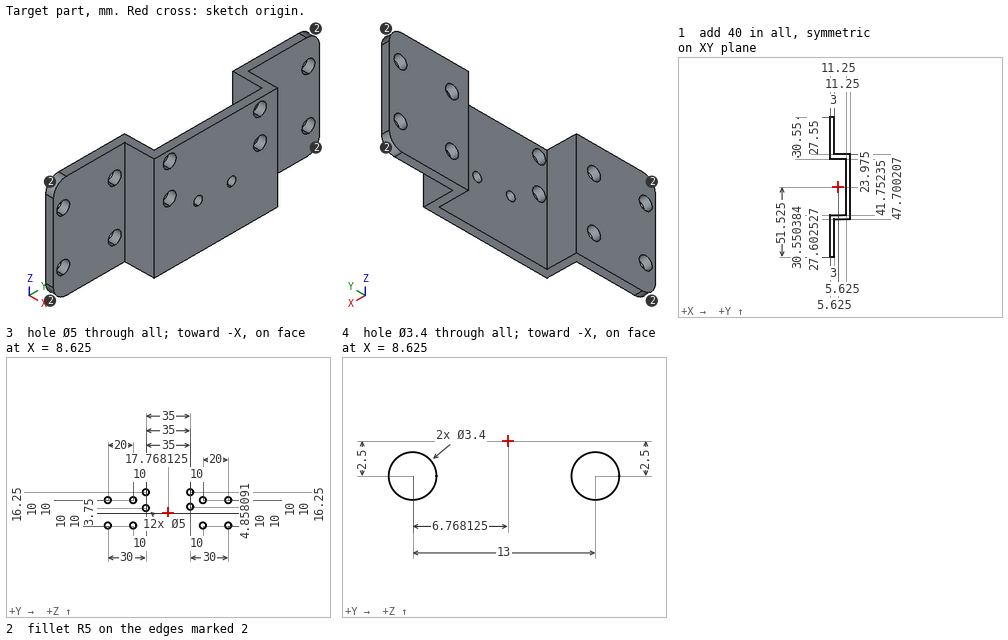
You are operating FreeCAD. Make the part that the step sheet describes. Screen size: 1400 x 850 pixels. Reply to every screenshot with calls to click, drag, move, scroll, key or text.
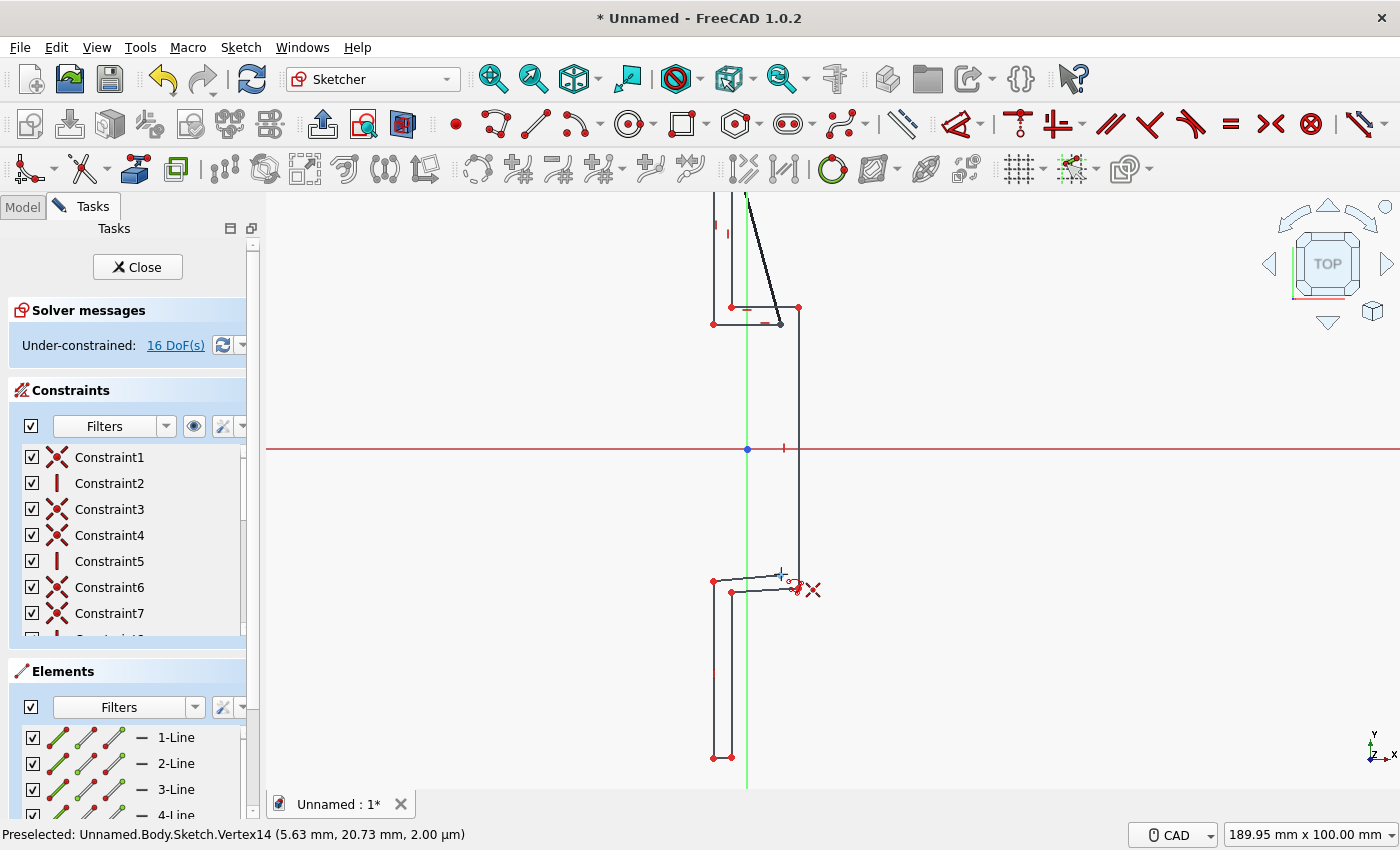
click(781, 575)
key(Escape)
key(Escape)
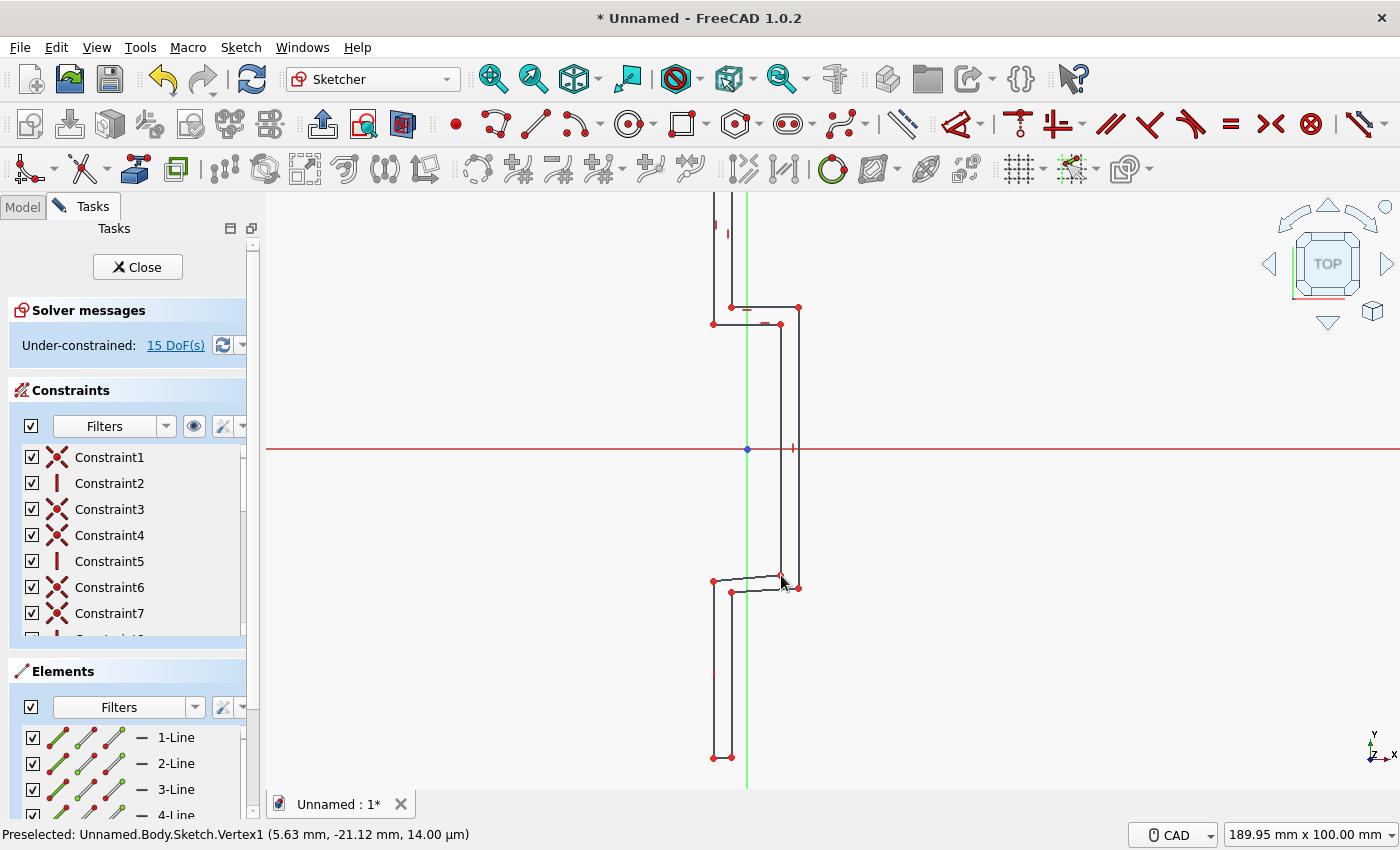
scroll(723, 758, up, 3)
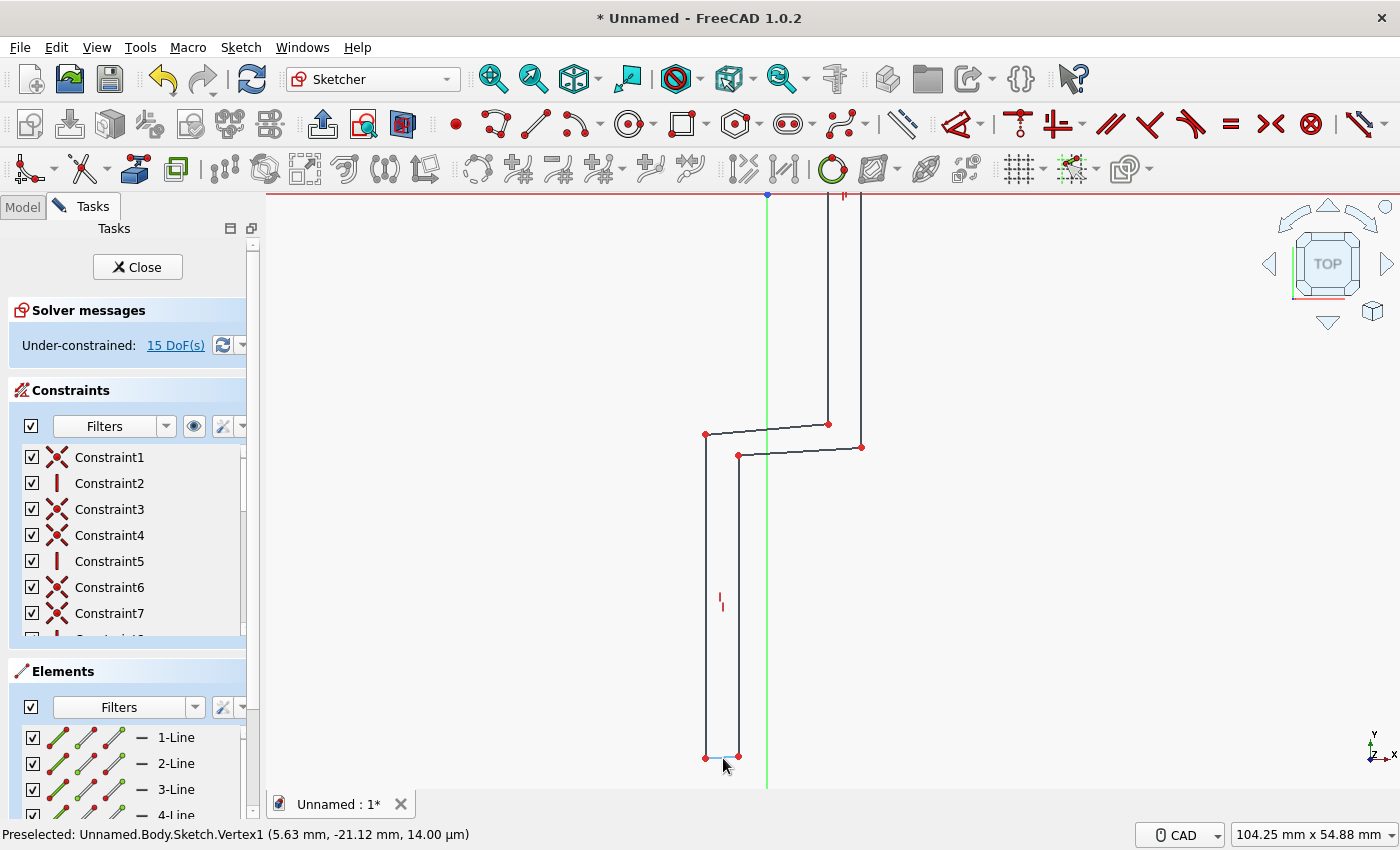
click(722, 758)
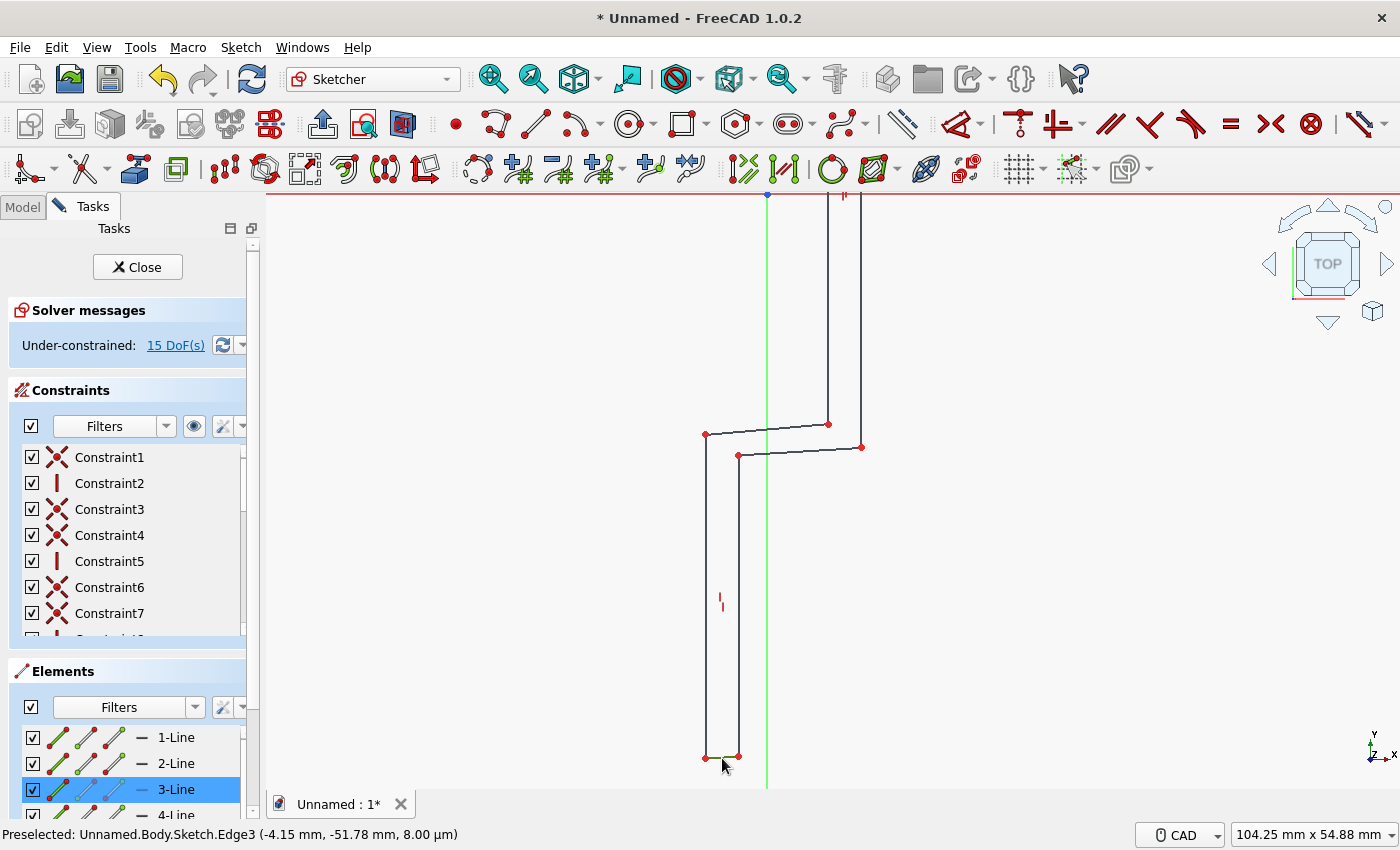
click(1084, 124)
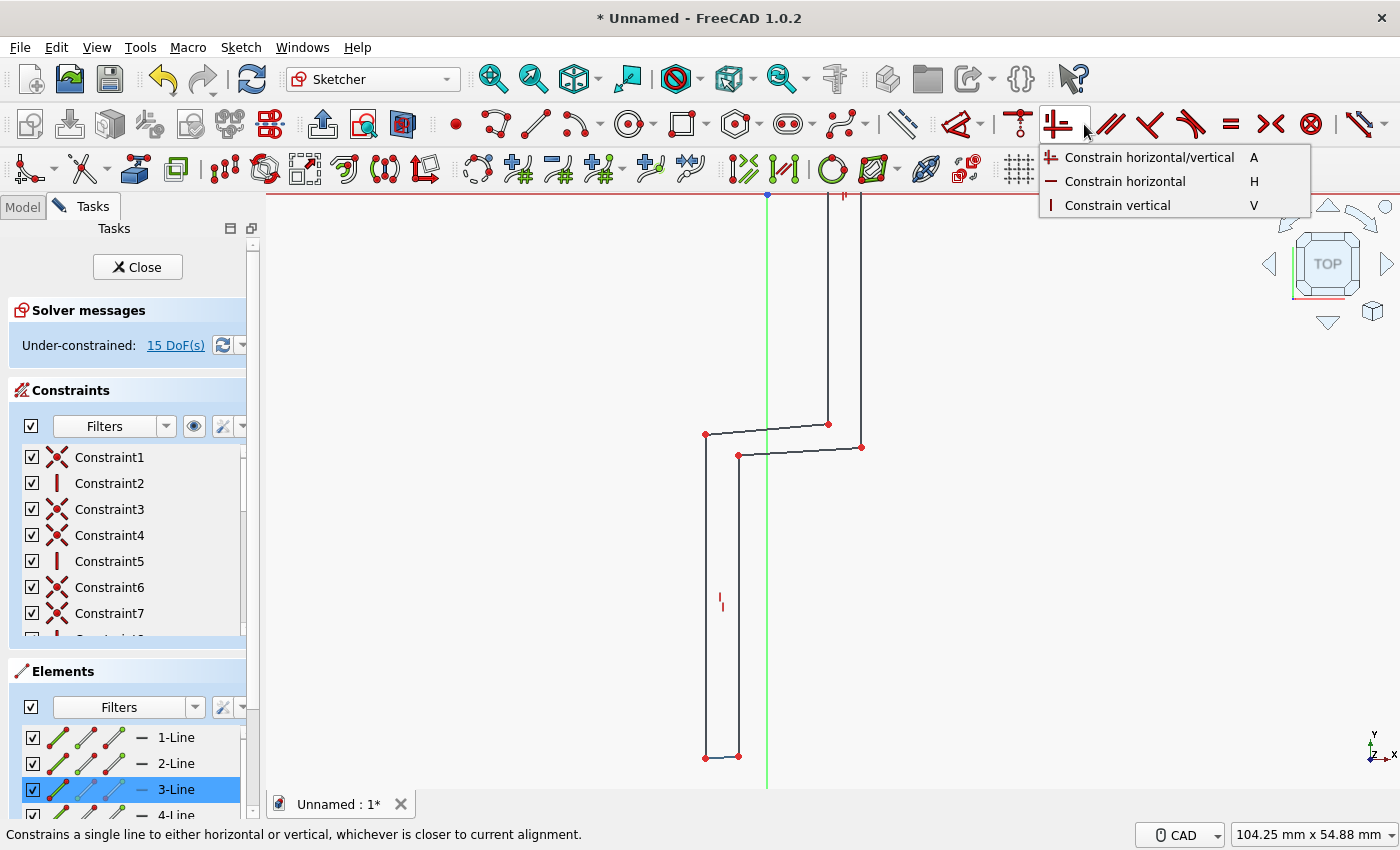
click(1175, 181)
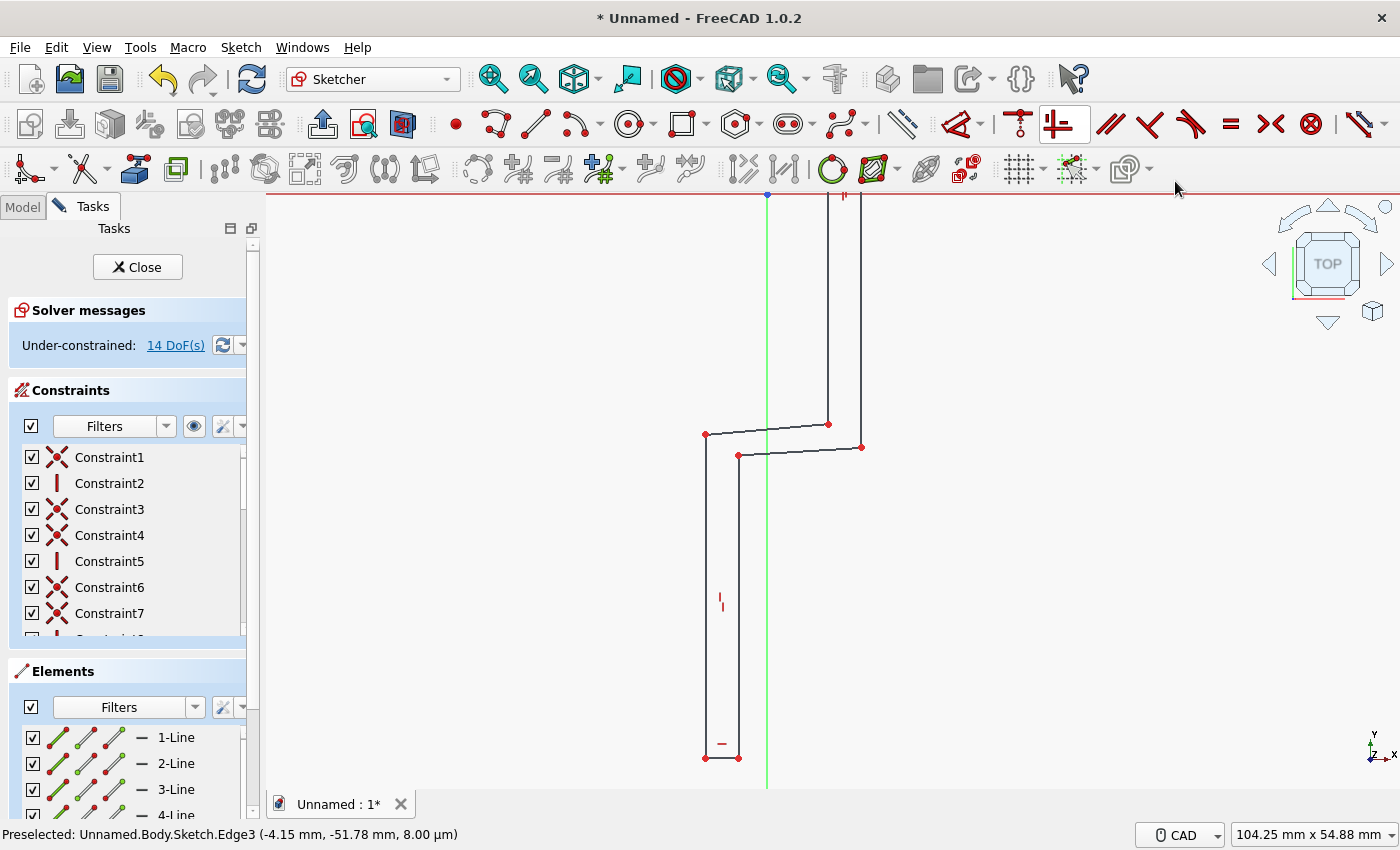
click(956, 124)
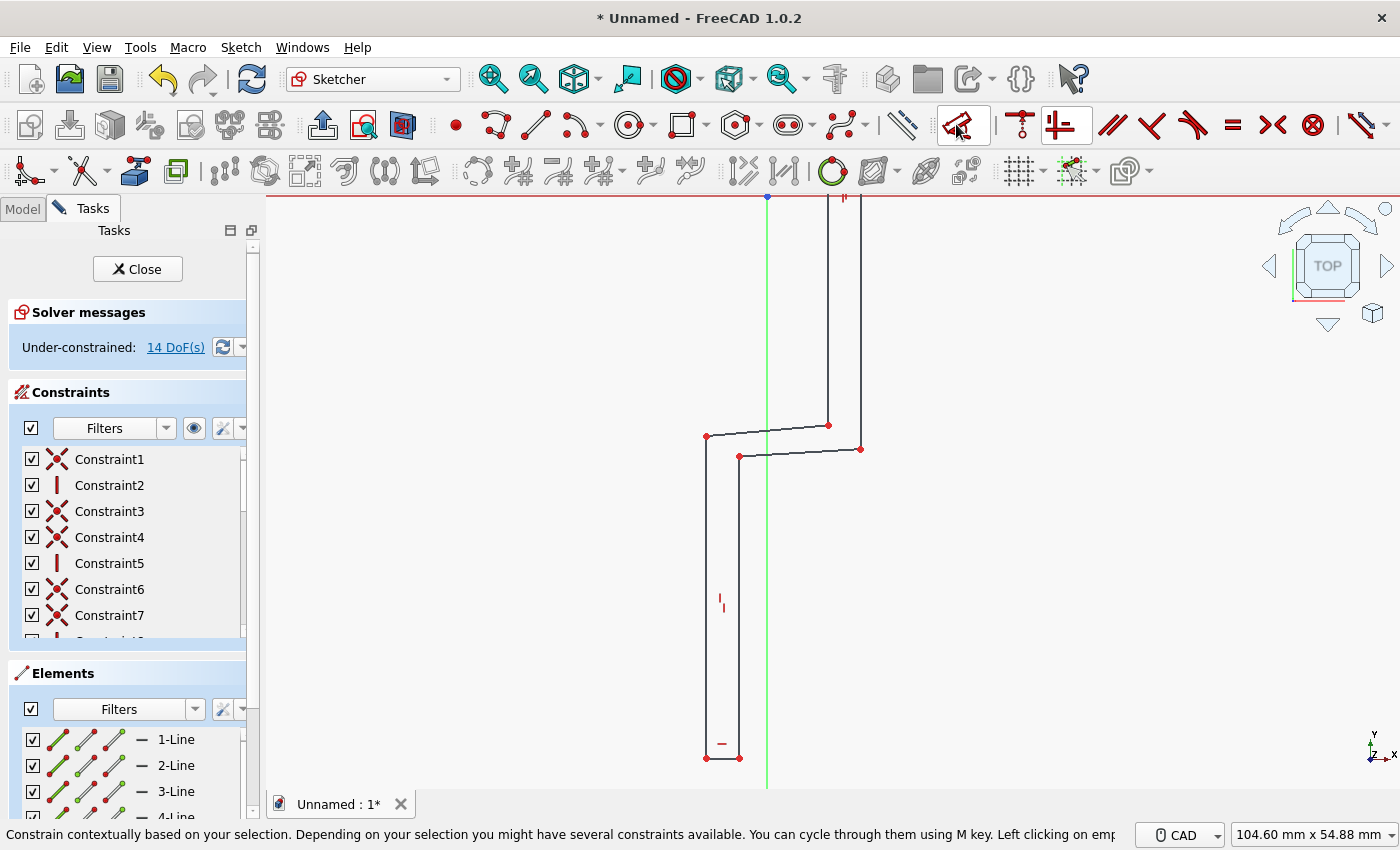
scroll(716, 759, up, 2)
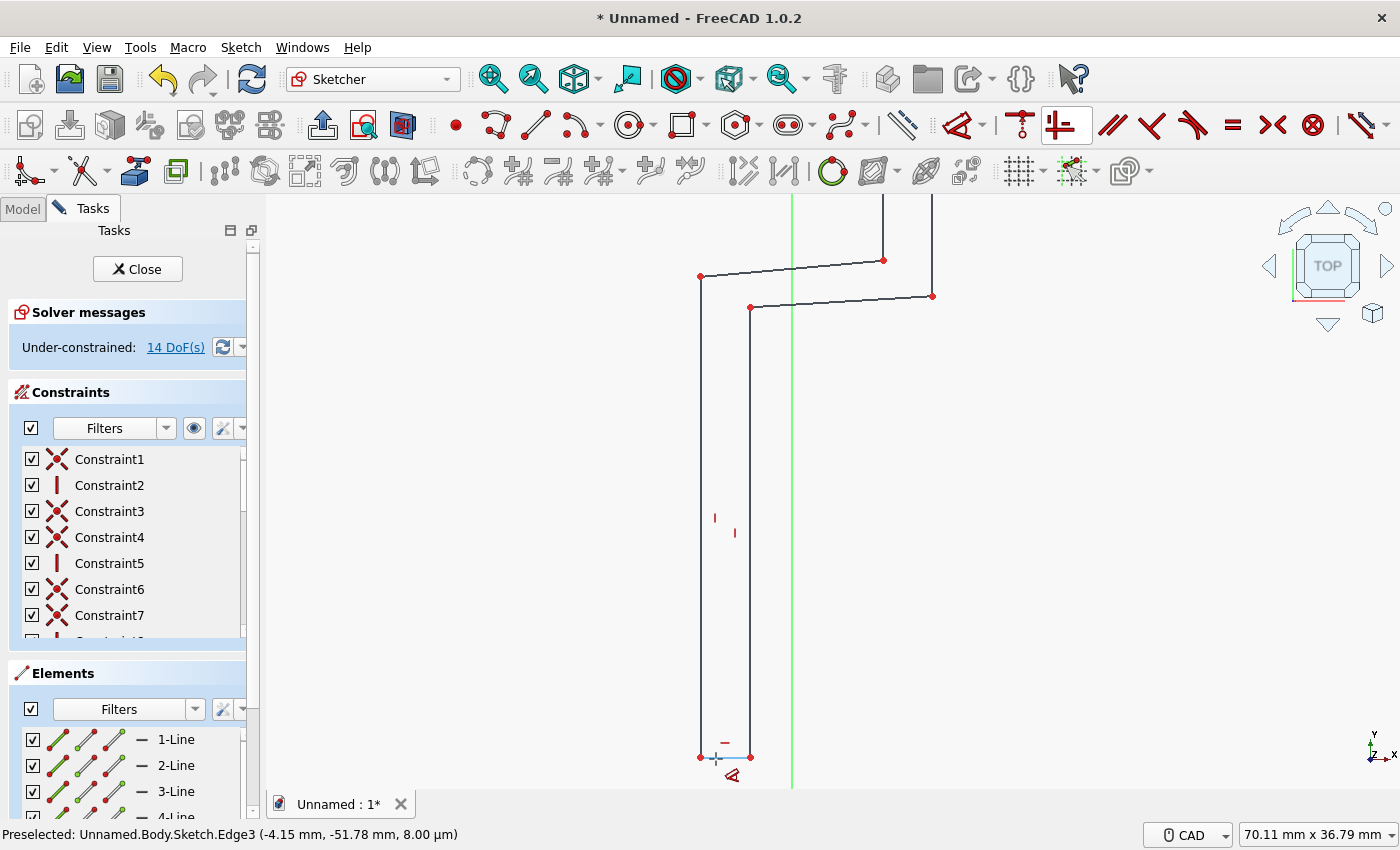
click(716, 758)
click(726, 724)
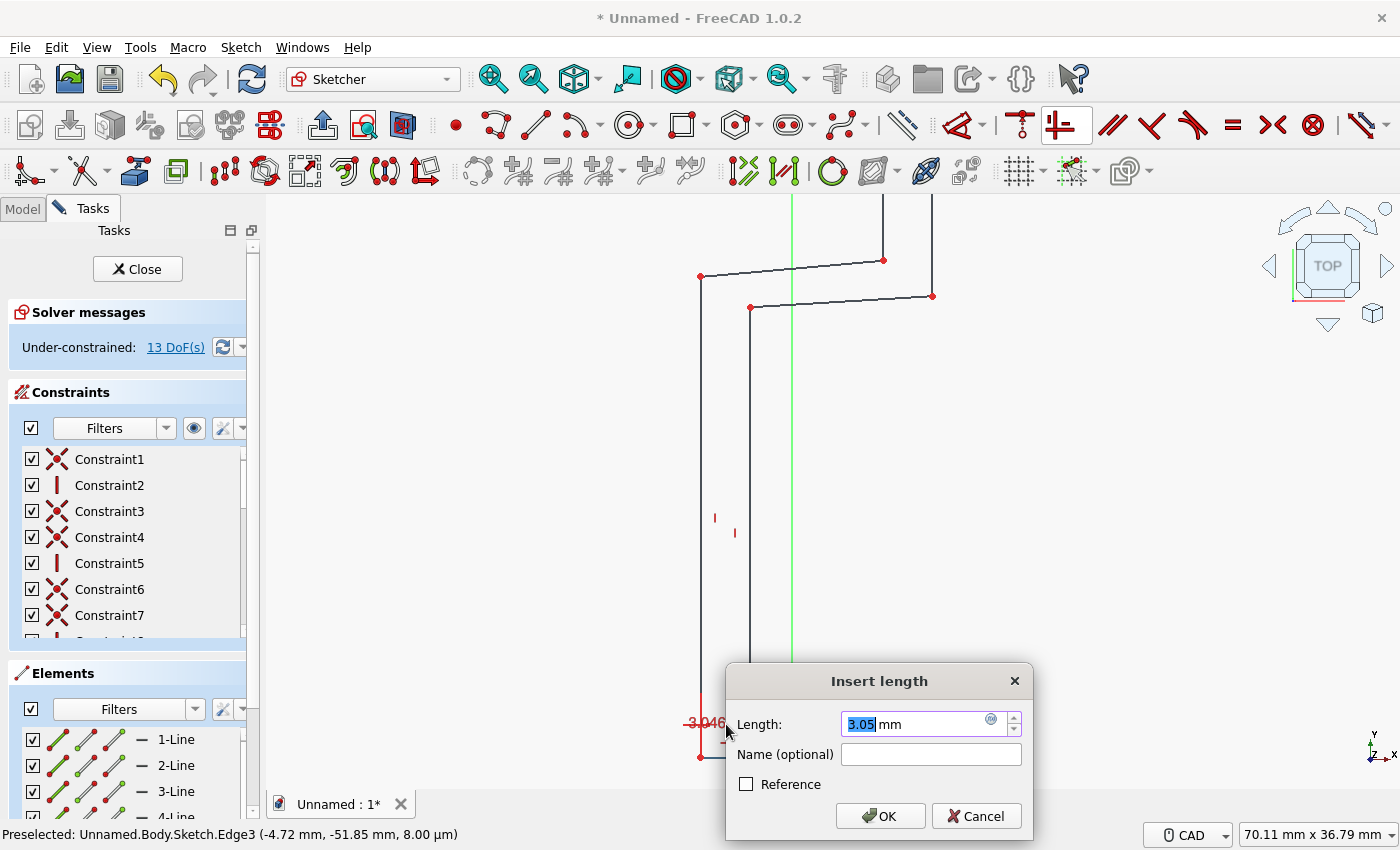
text(3)
key(Return)